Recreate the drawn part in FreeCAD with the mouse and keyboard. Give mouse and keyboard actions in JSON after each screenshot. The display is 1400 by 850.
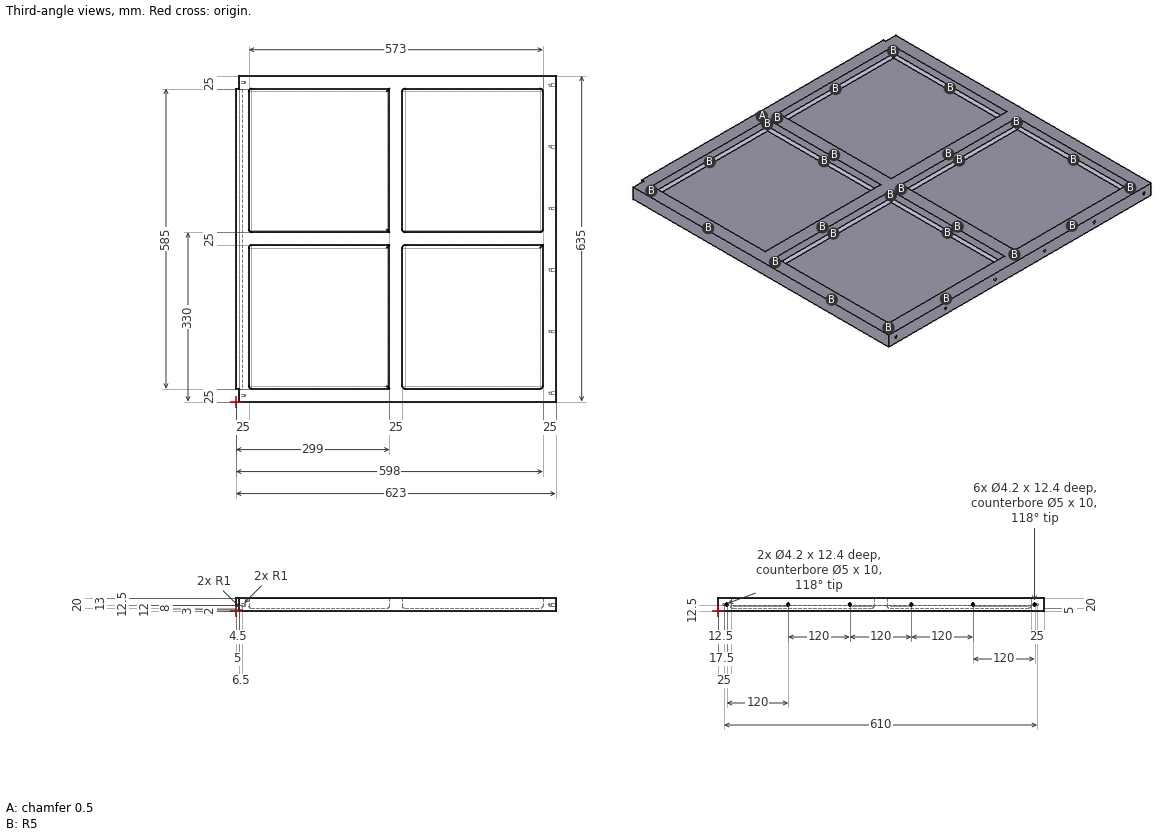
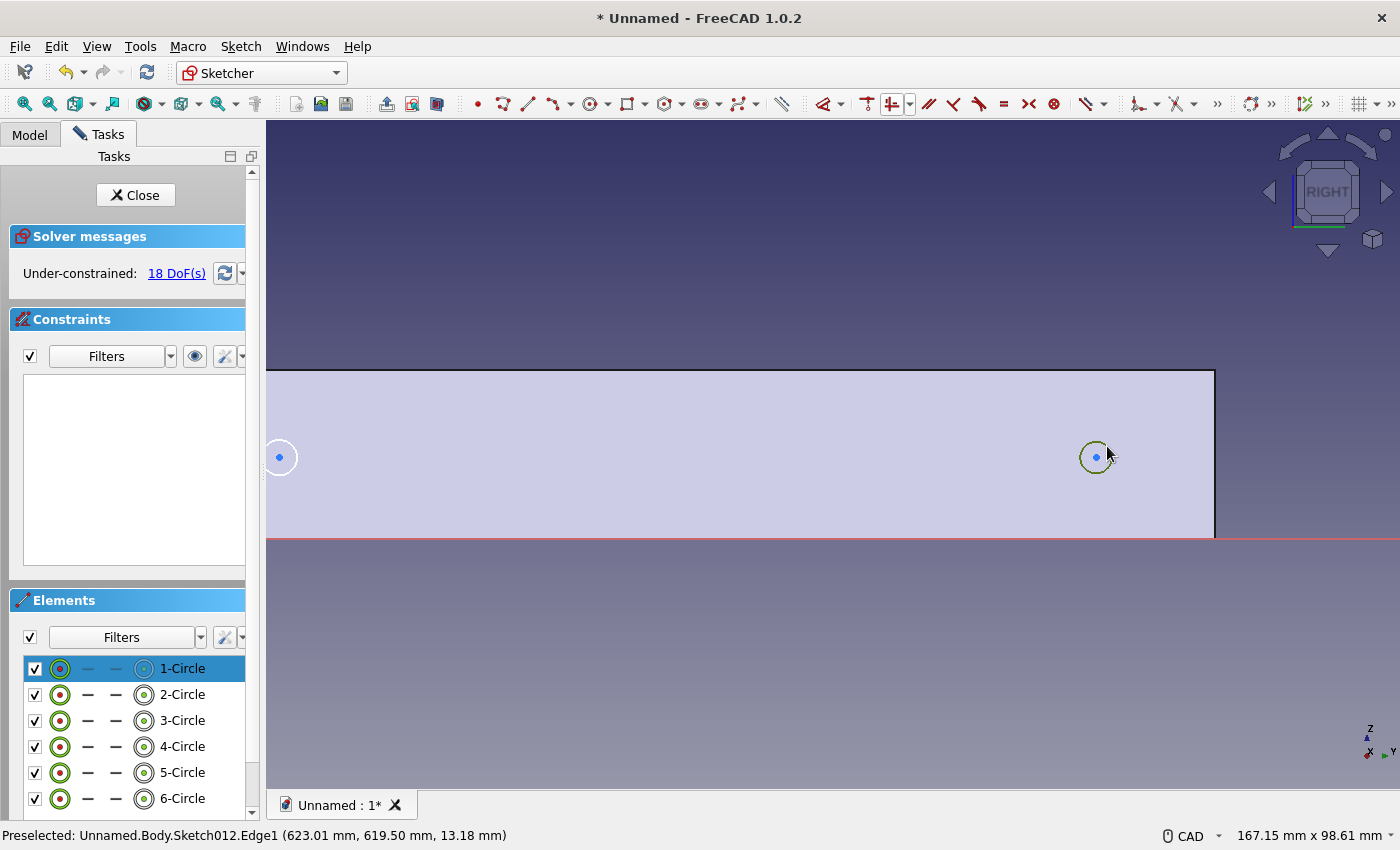
{"action": "left_click", "coordinate": [297, 458]}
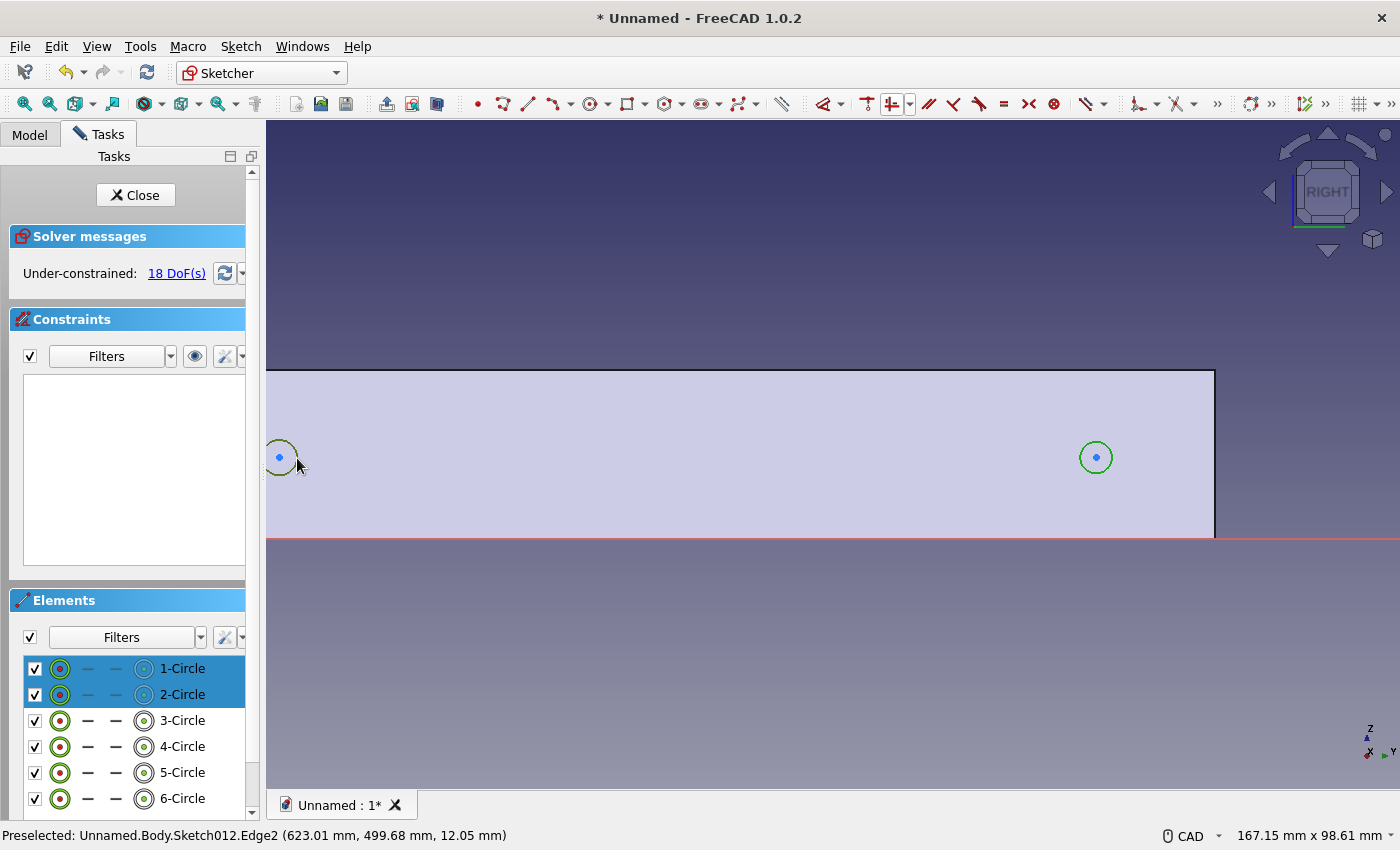
{"action": "scroll", "coordinate": [1112, 447], "scroll_direction": "down", "scroll_amount": 9}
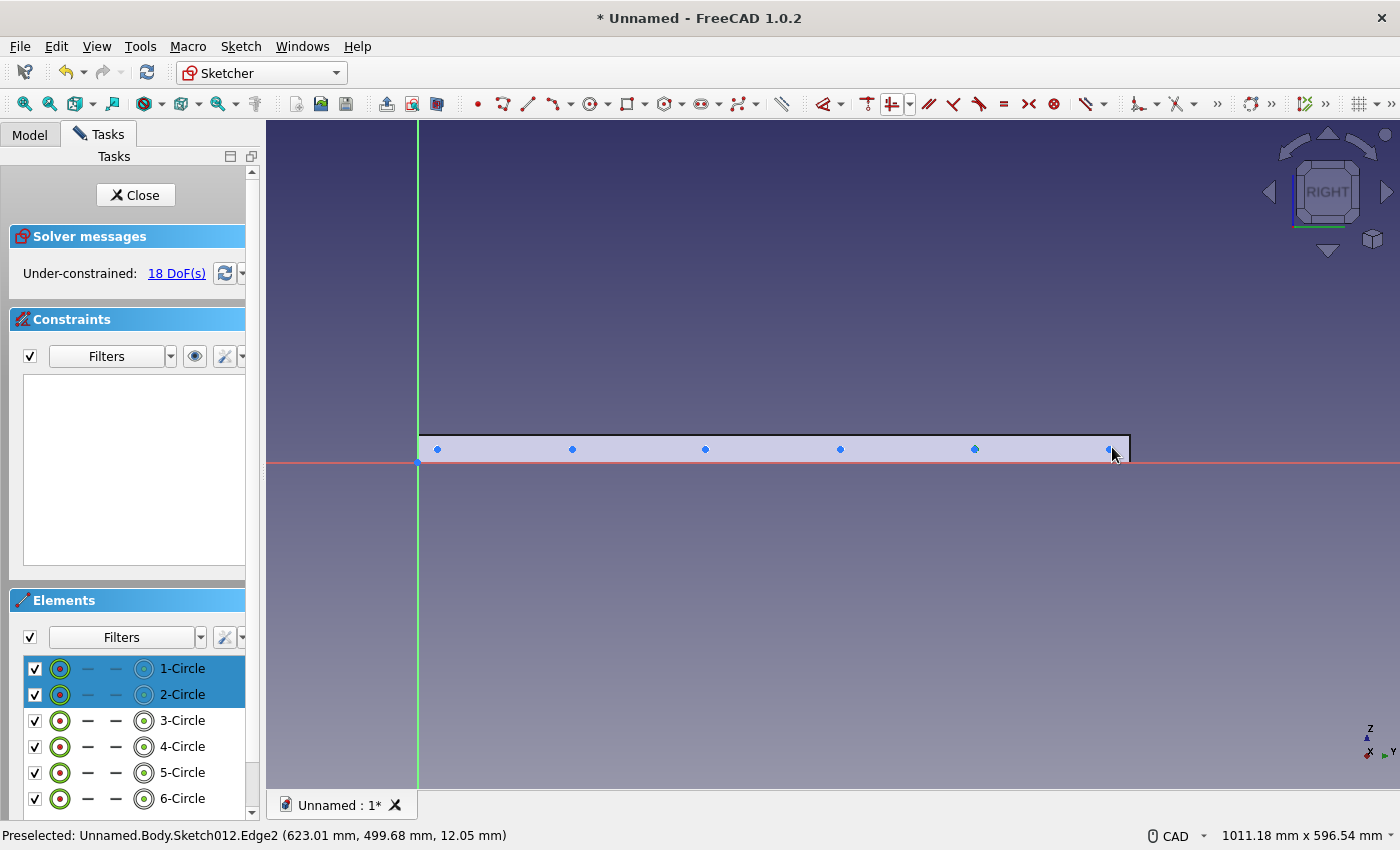
{"action": "scroll", "coordinate": [843, 447], "scroll_direction": "up", "scroll_amount": 9}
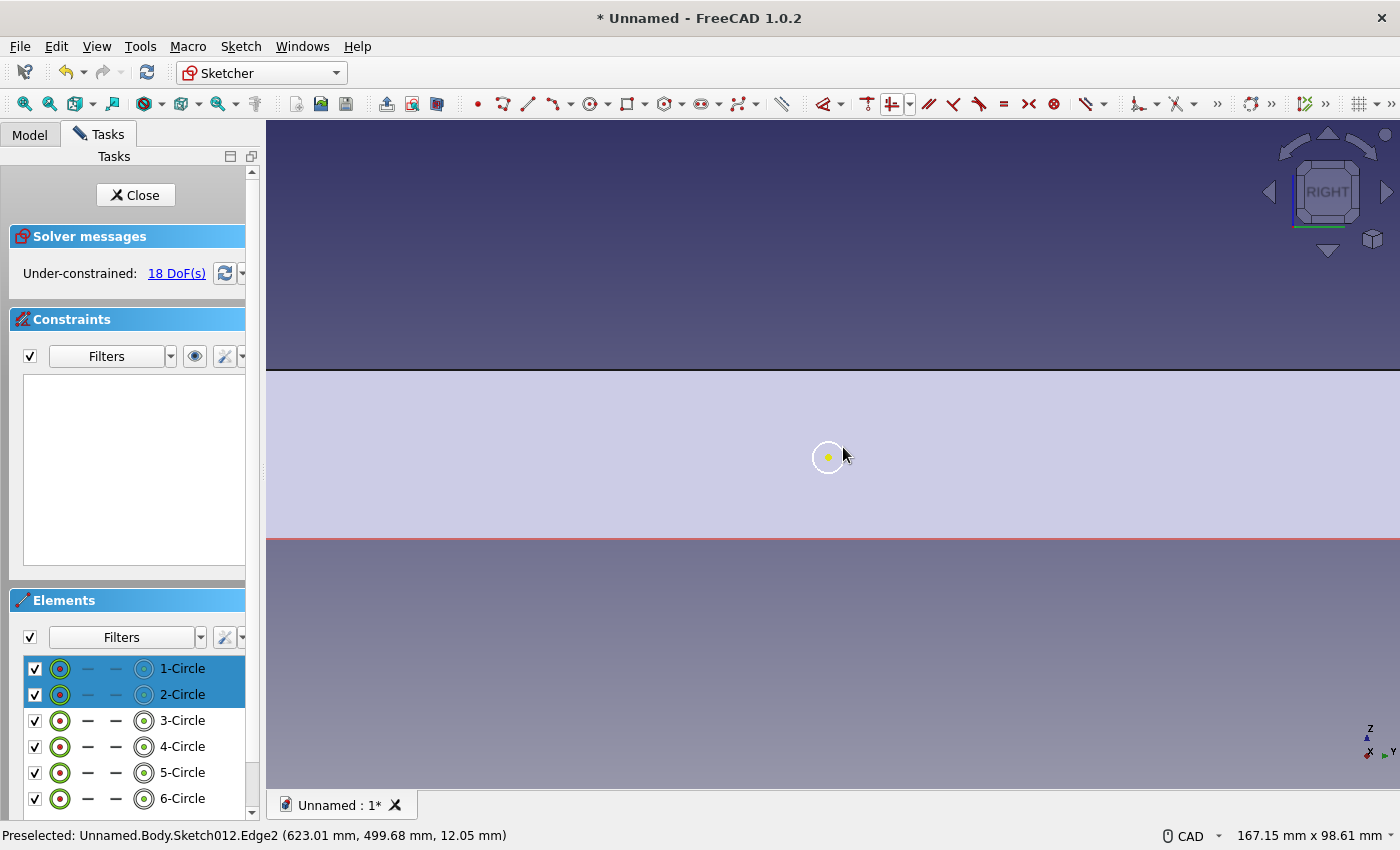
{"action": "left_click", "coordinate": [839, 447]}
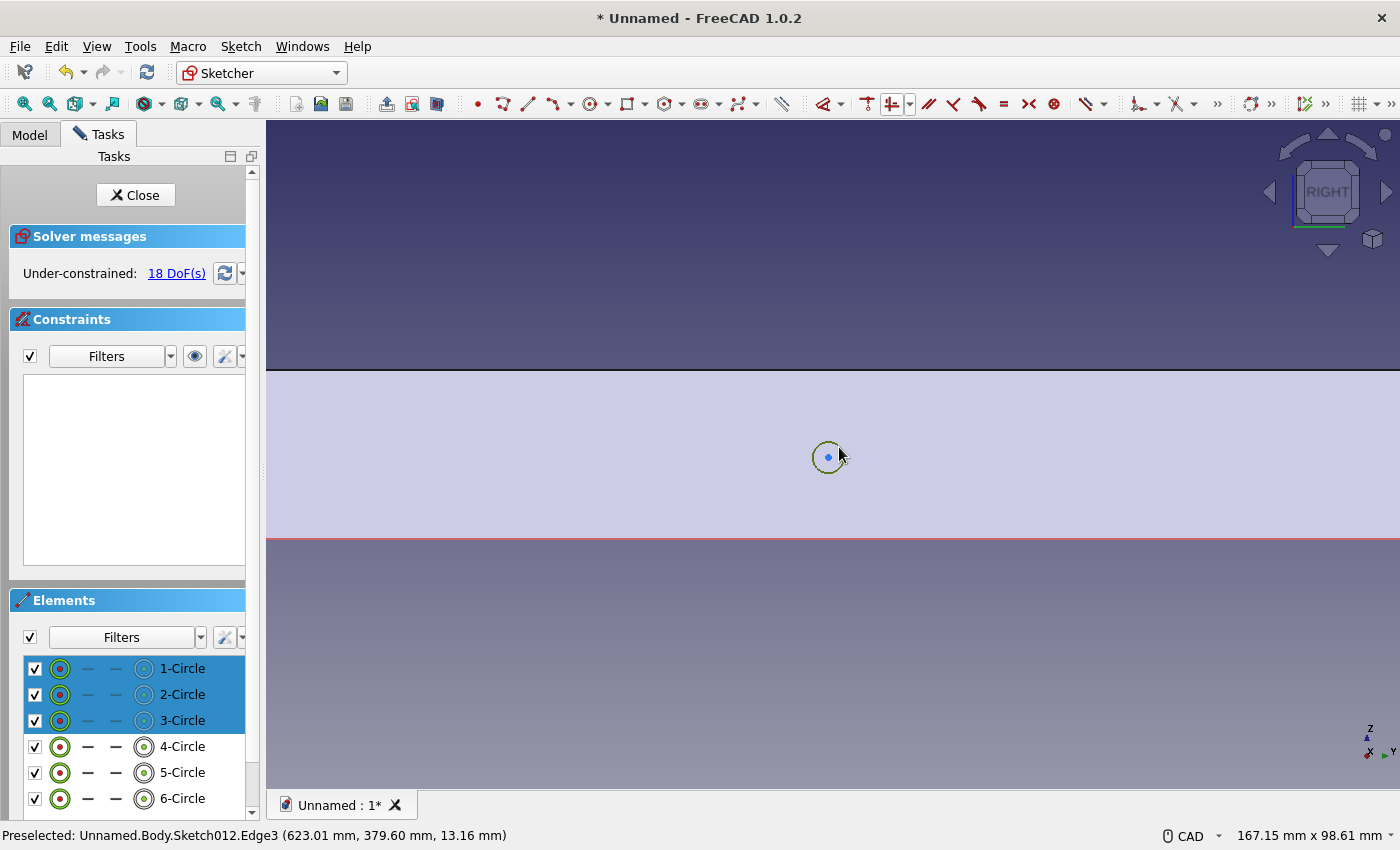
{"action": "scroll", "coordinate": [843, 447], "scroll_direction": "down", "scroll_amount": 9}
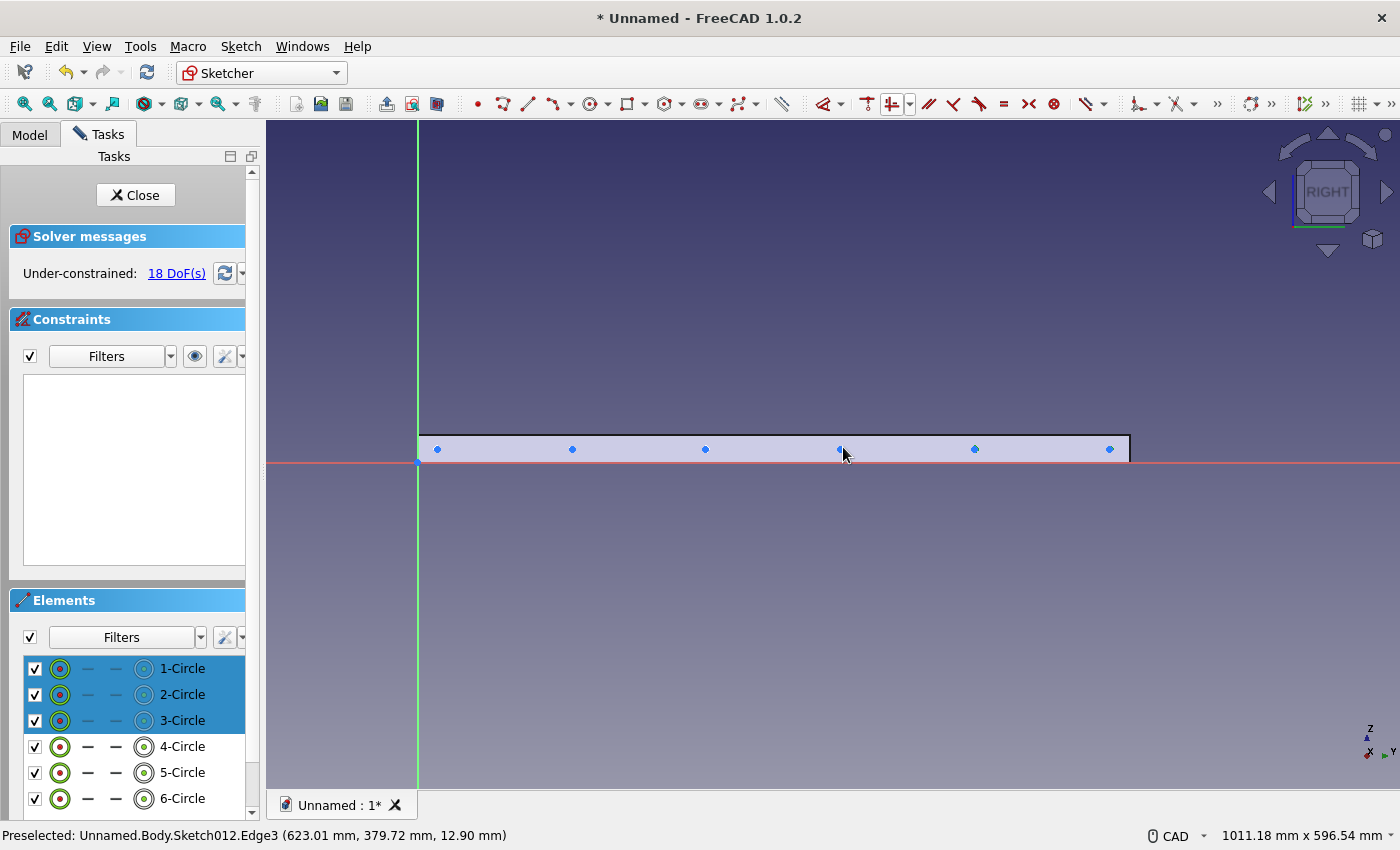
{"action": "scroll", "coordinate": [708, 447], "scroll_direction": "up", "scroll_amount": 9}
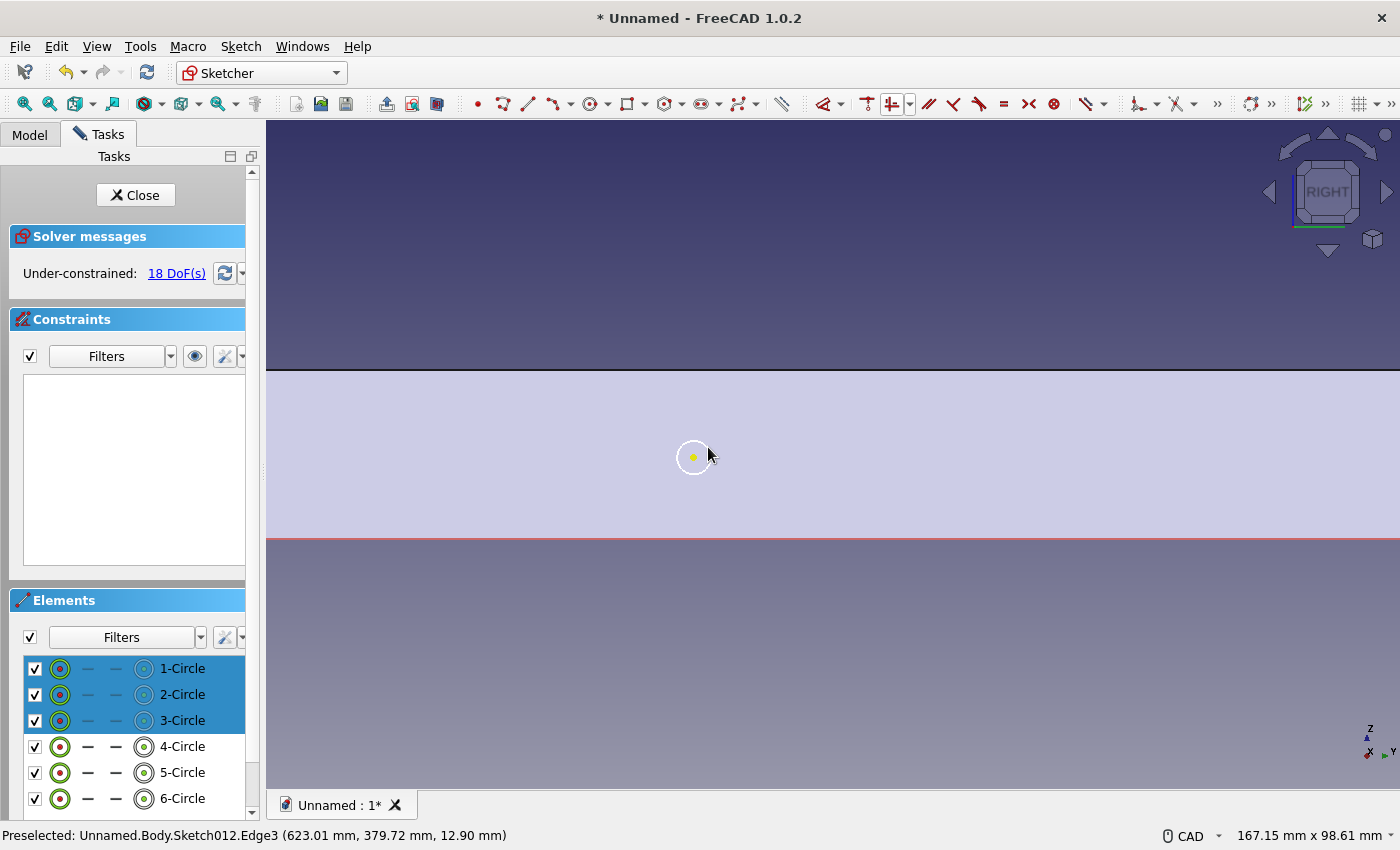
{"action": "left_click", "coordinate": [706, 446]}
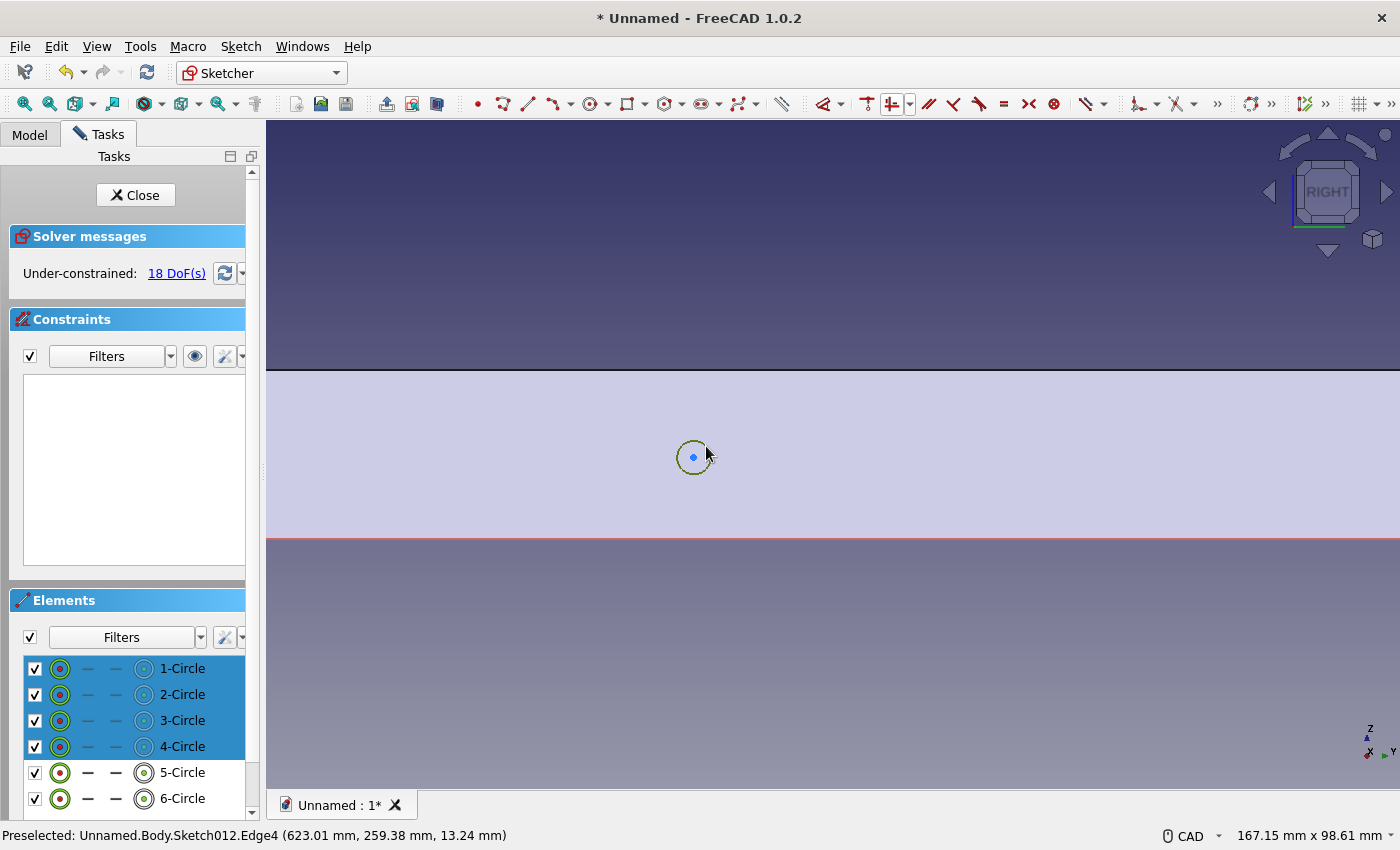
{"action": "scroll", "coordinate": [708, 447], "scroll_direction": "down", "scroll_amount": 9}